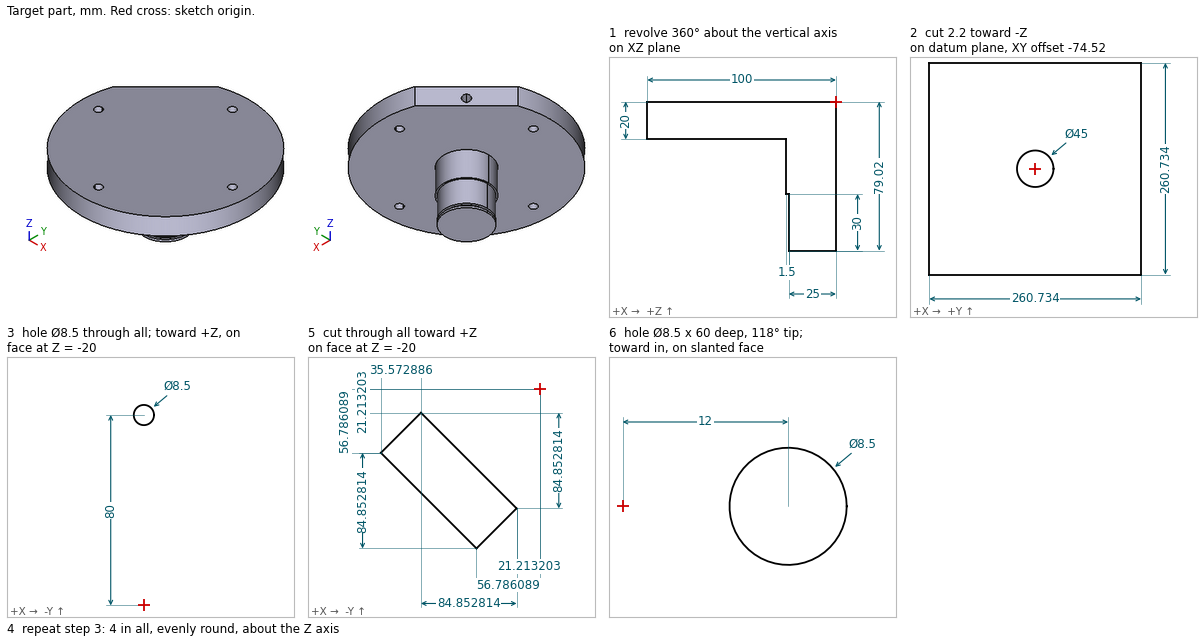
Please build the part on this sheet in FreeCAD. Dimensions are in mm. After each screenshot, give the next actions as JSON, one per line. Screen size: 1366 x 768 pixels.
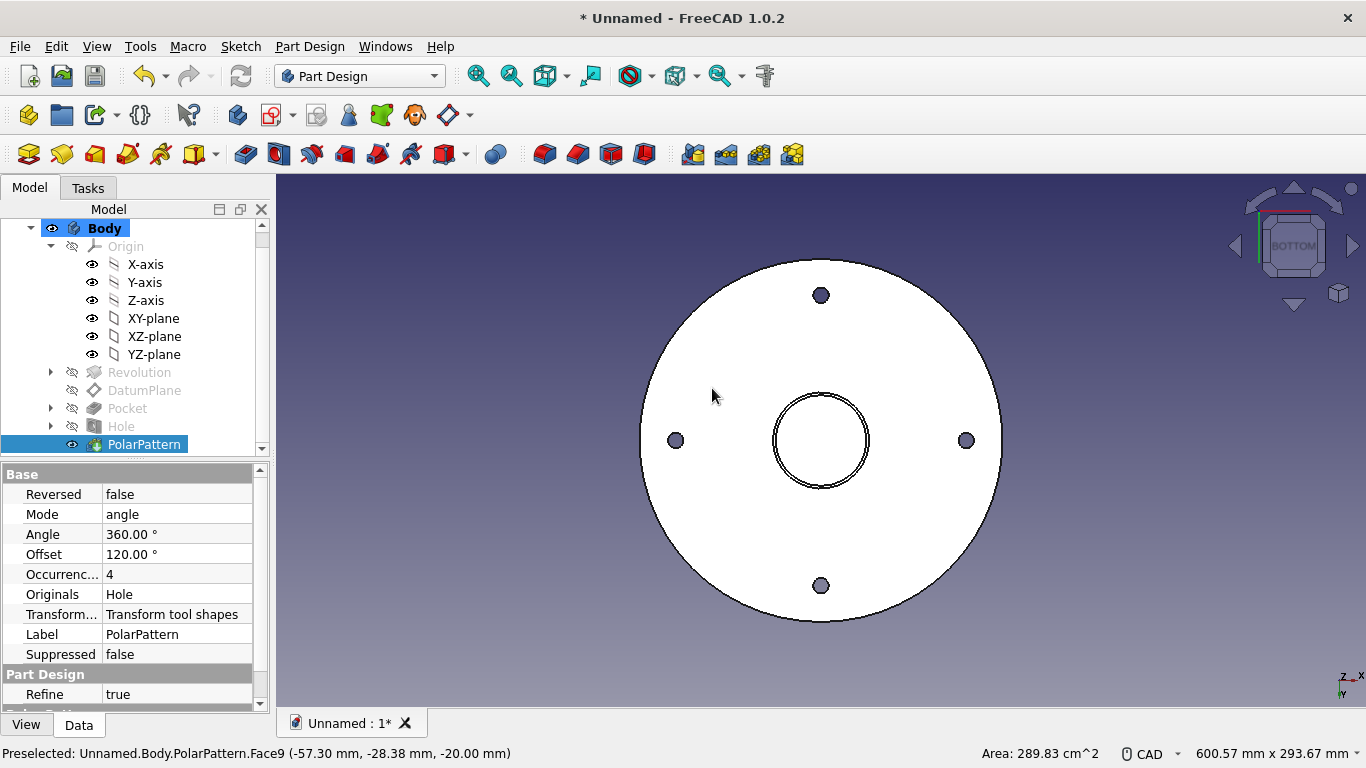
{"action": "left_click", "coordinate": [270, 116]}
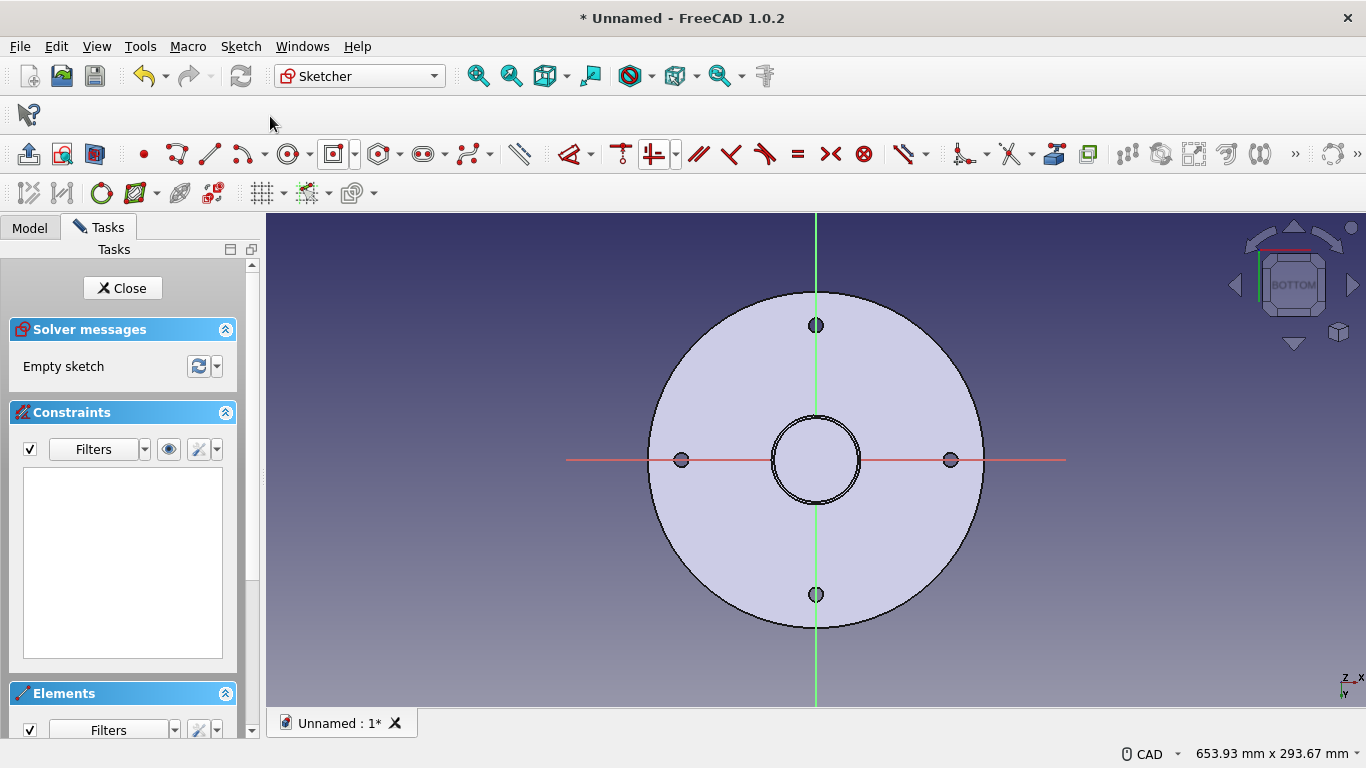
{"action": "scroll", "coordinate": [976, 241], "scroll_direction": "down", "scroll_amount": 1}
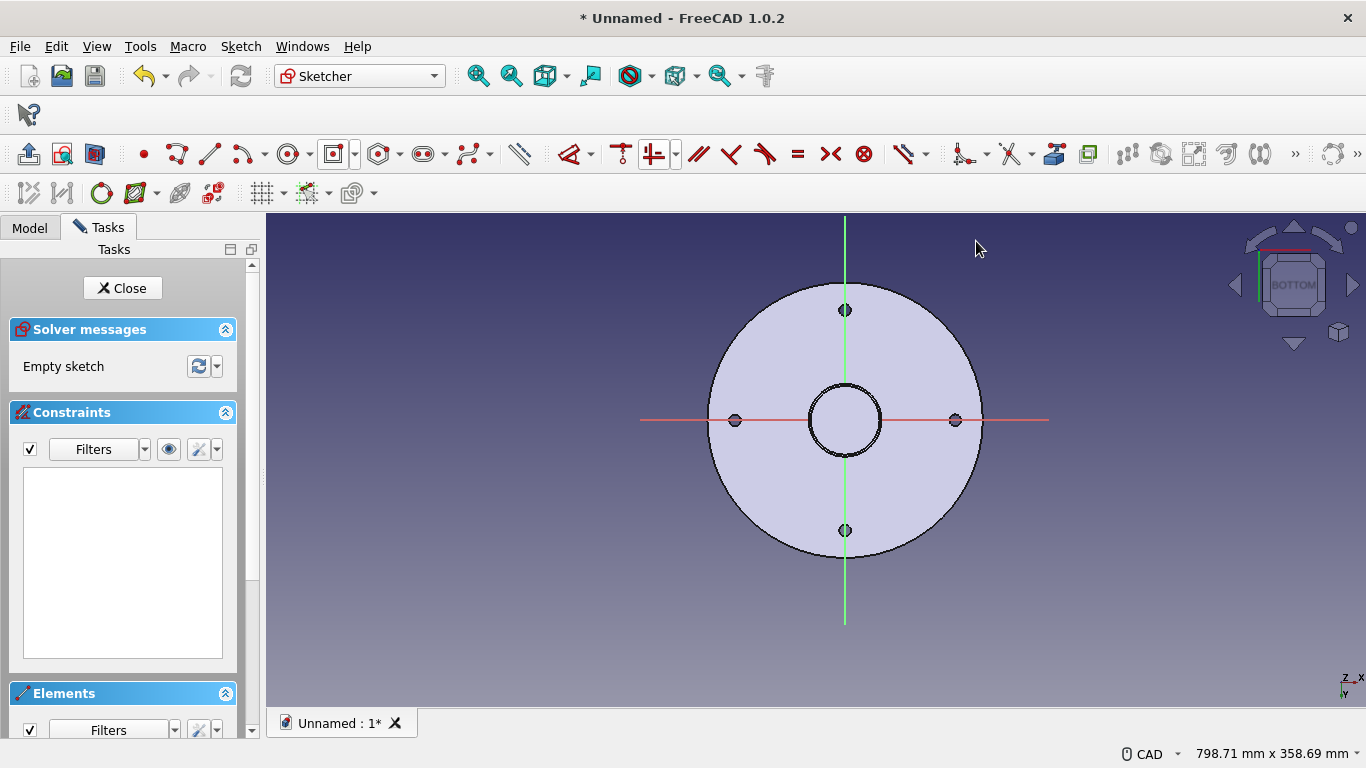
{"action": "scroll", "coordinate": [748, 635], "scroll_direction": "up", "scroll_amount": 2}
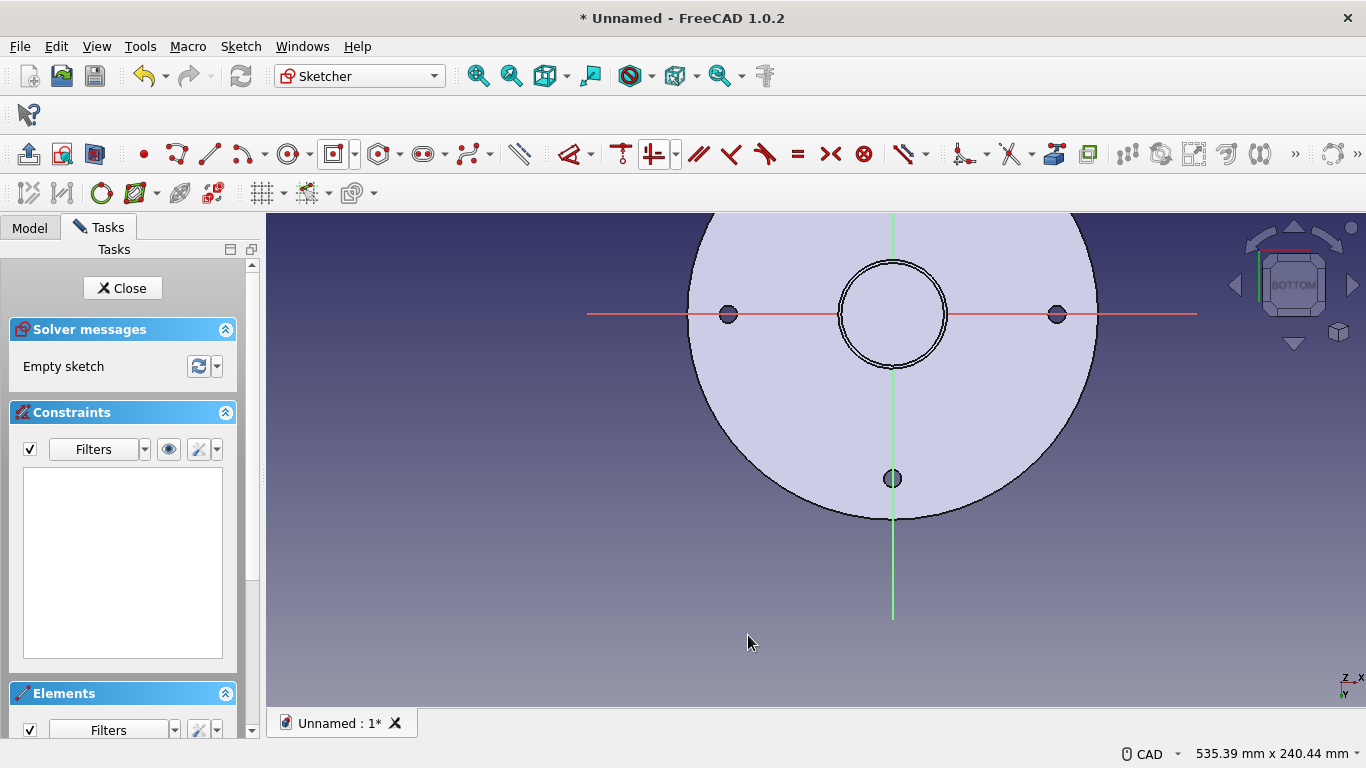
{"action": "left_click", "coordinate": [177, 154]}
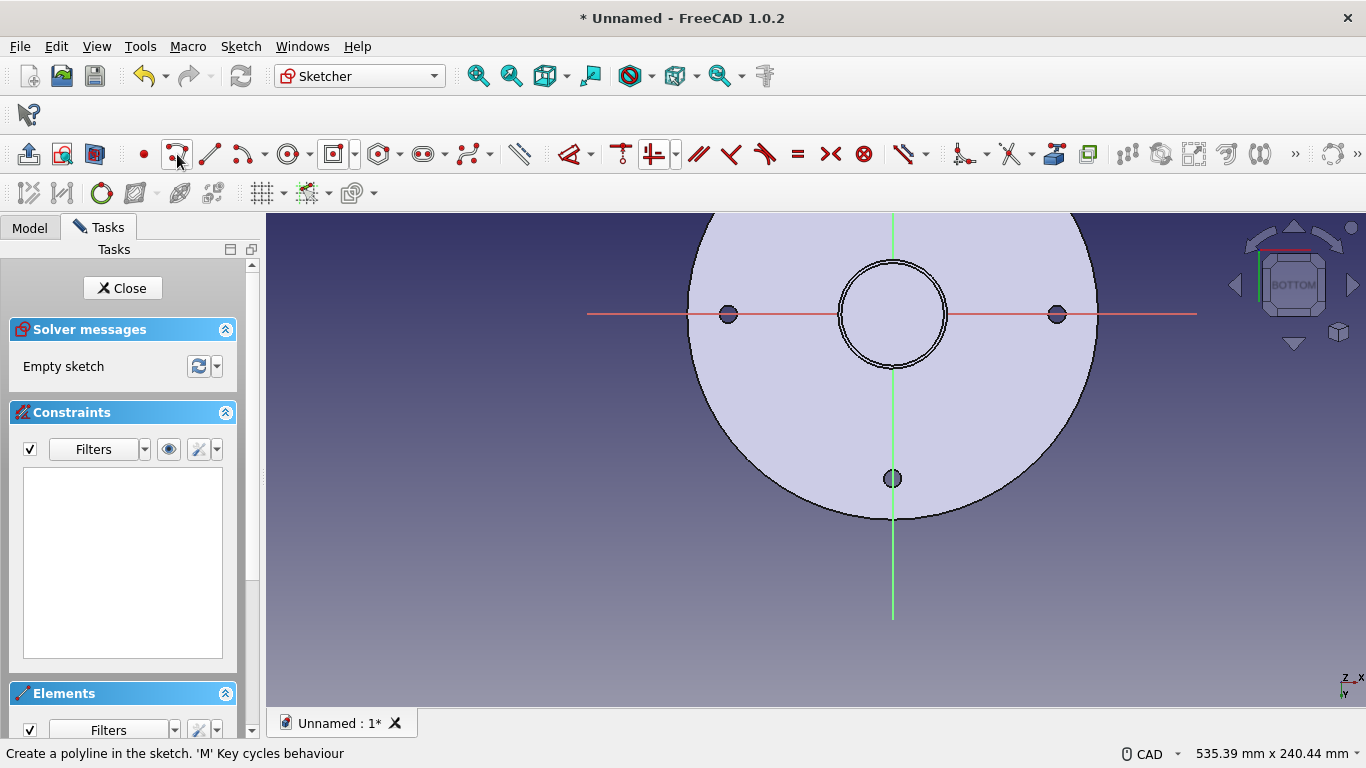
{"action": "left_click", "coordinate": [849, 532]}
{"action": "left_click", "coordinate": [675, 358]}
{"action": "left_click", "coordinate": [602, 431]}
{"action": "left_click", "coordinate": [776, 605]}
{"action": "left_click", "coordinate": [849, 533]}
{"action": "key", "text": "Escape"}
{"action": "key", "text": "Escape"}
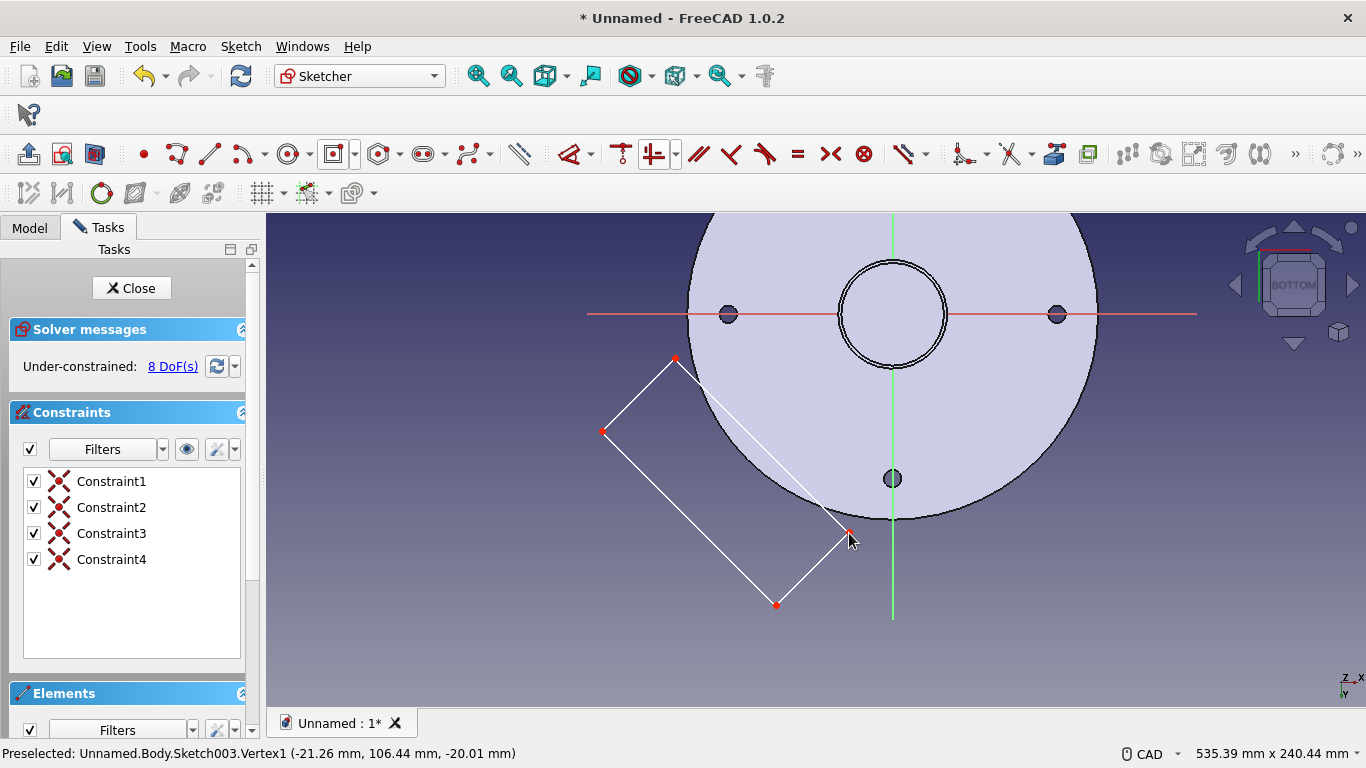
{"action": "left_click", "coordinate": [568, 154]}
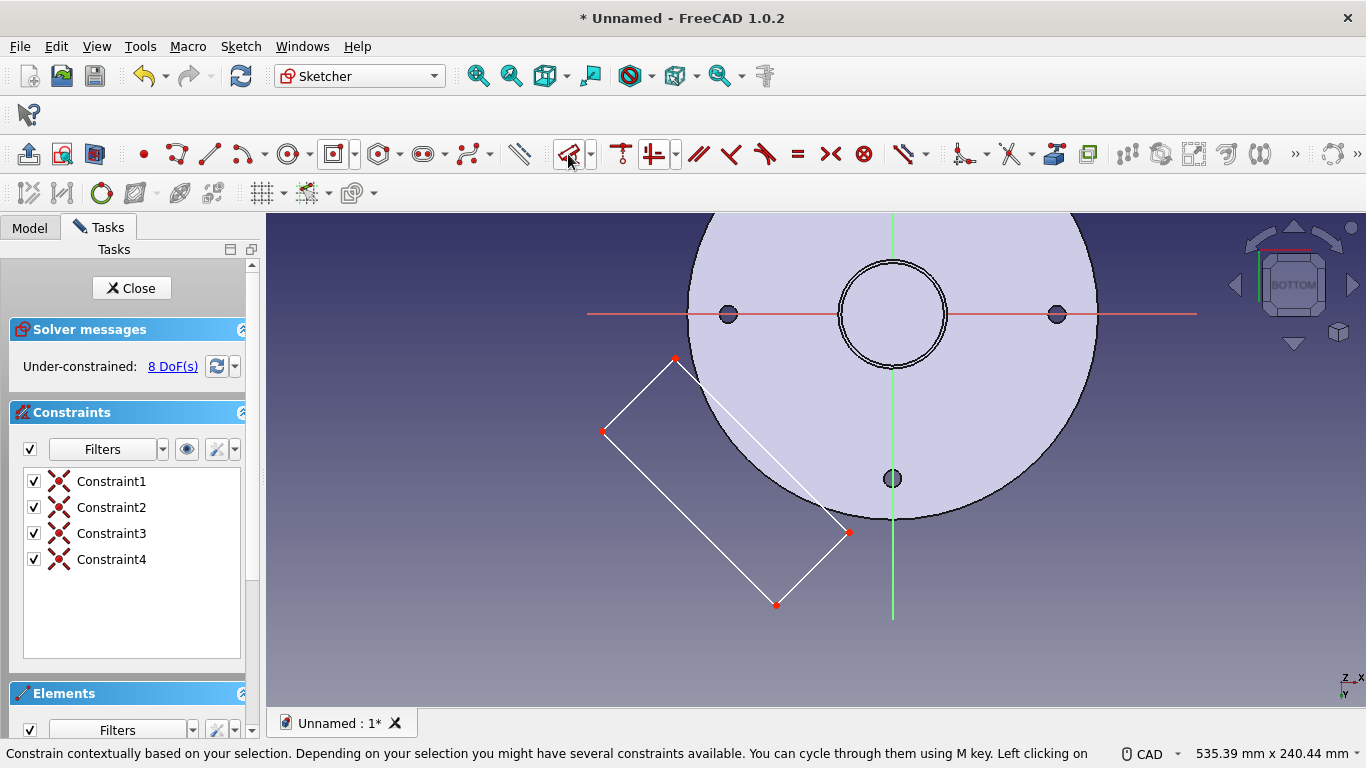
{"action": "left_click", "coordinate": [849, 533]}
{"action": "left_click", "coordinate": [871, 280]}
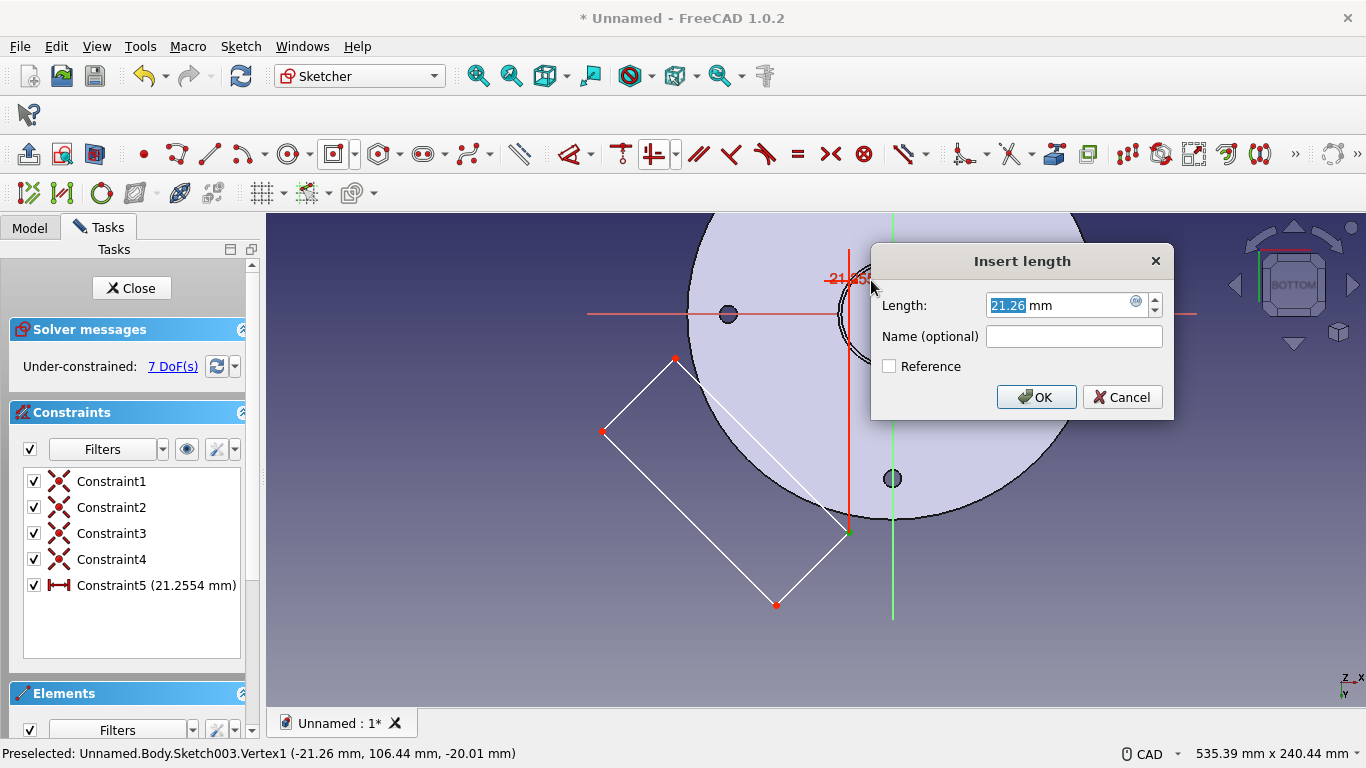
{"action": "type", "text": "21.213203"}
{"action": "key", "text": "Return"}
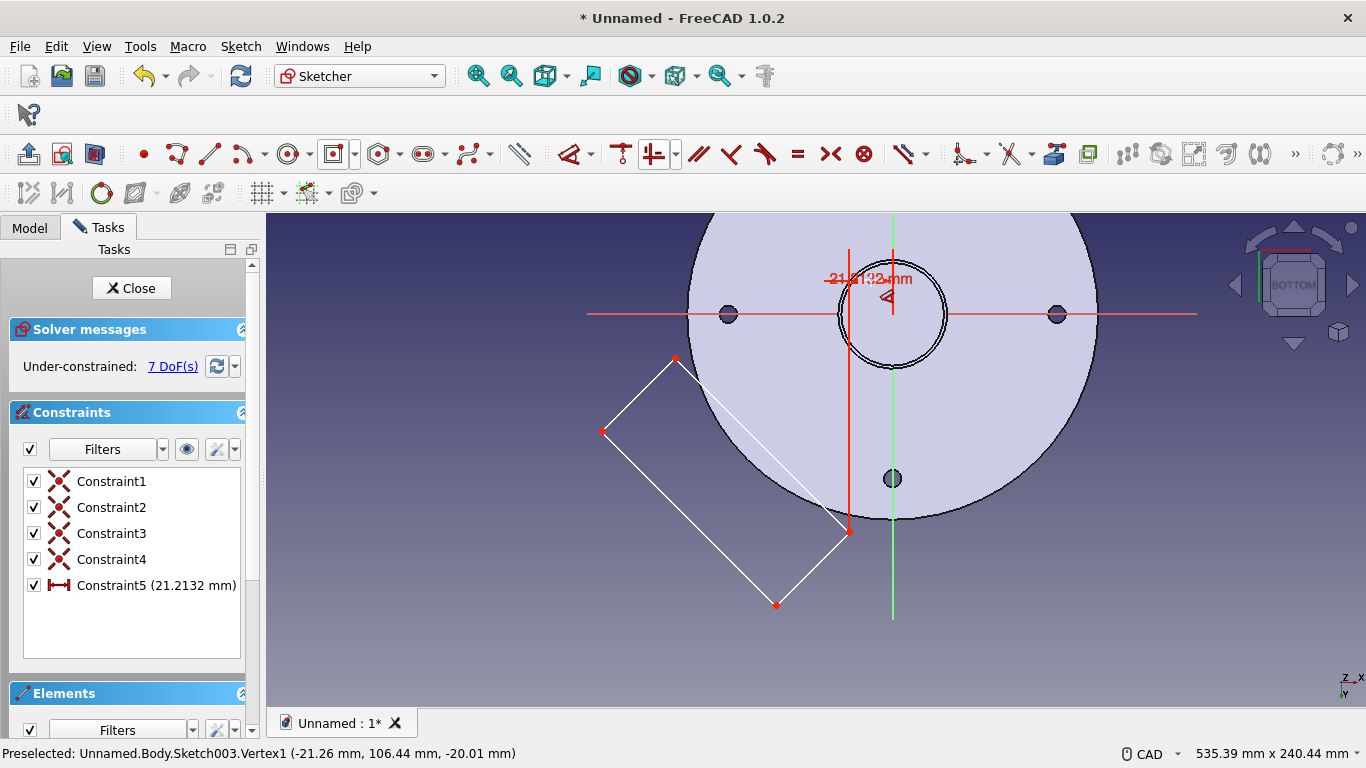
{"action": "left_click", "coordinate": [675, 359]}
{"action": "left_click", "coordinate": [927, 337]}